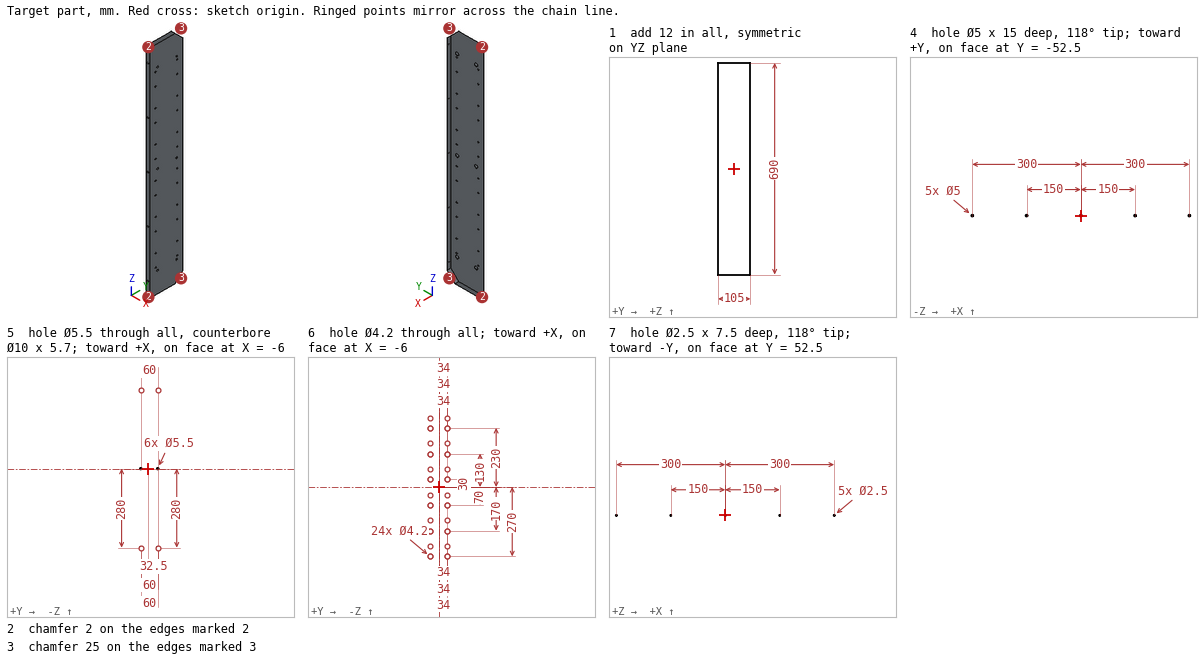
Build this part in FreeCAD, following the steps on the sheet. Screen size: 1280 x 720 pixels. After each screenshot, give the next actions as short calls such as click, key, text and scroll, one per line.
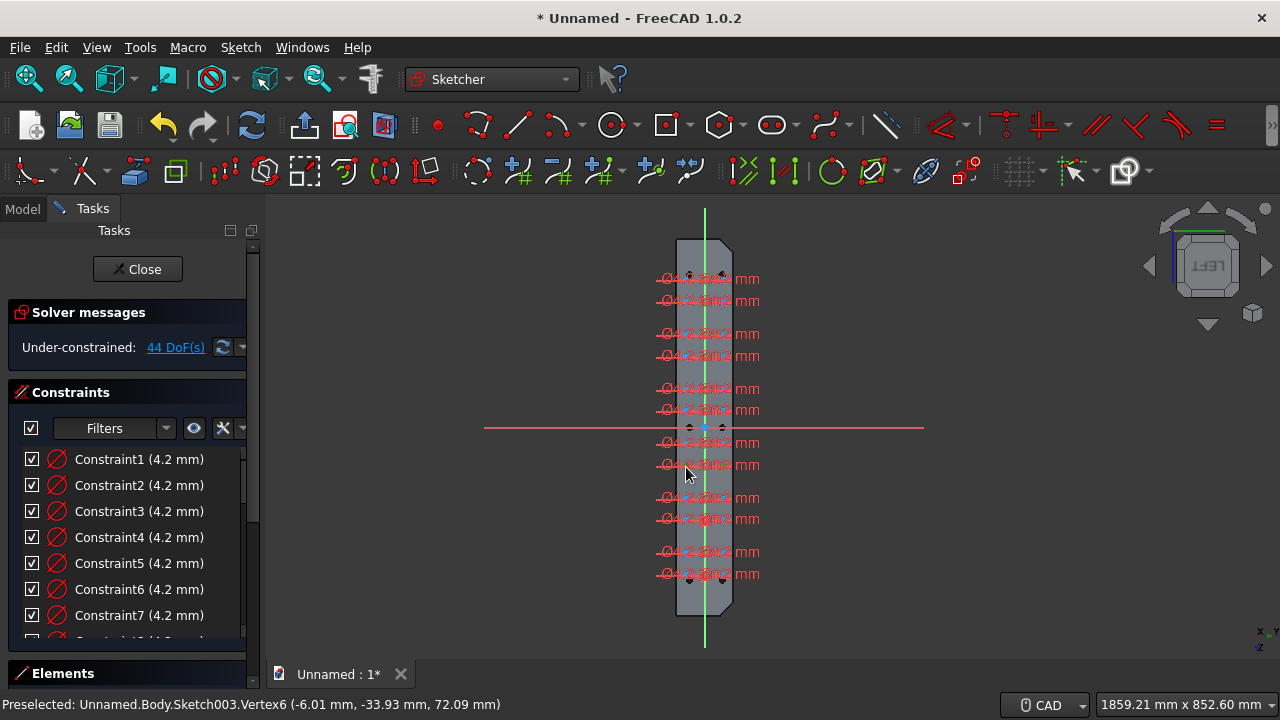
click(705, 602)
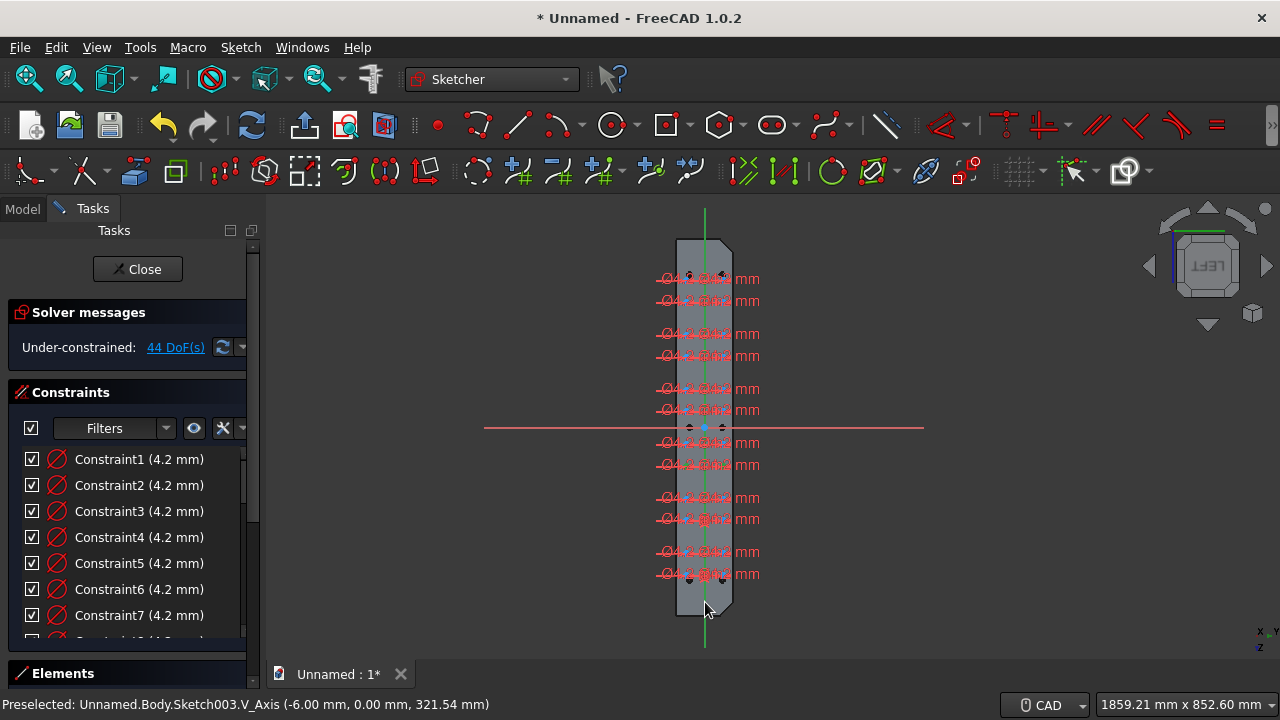
key(s)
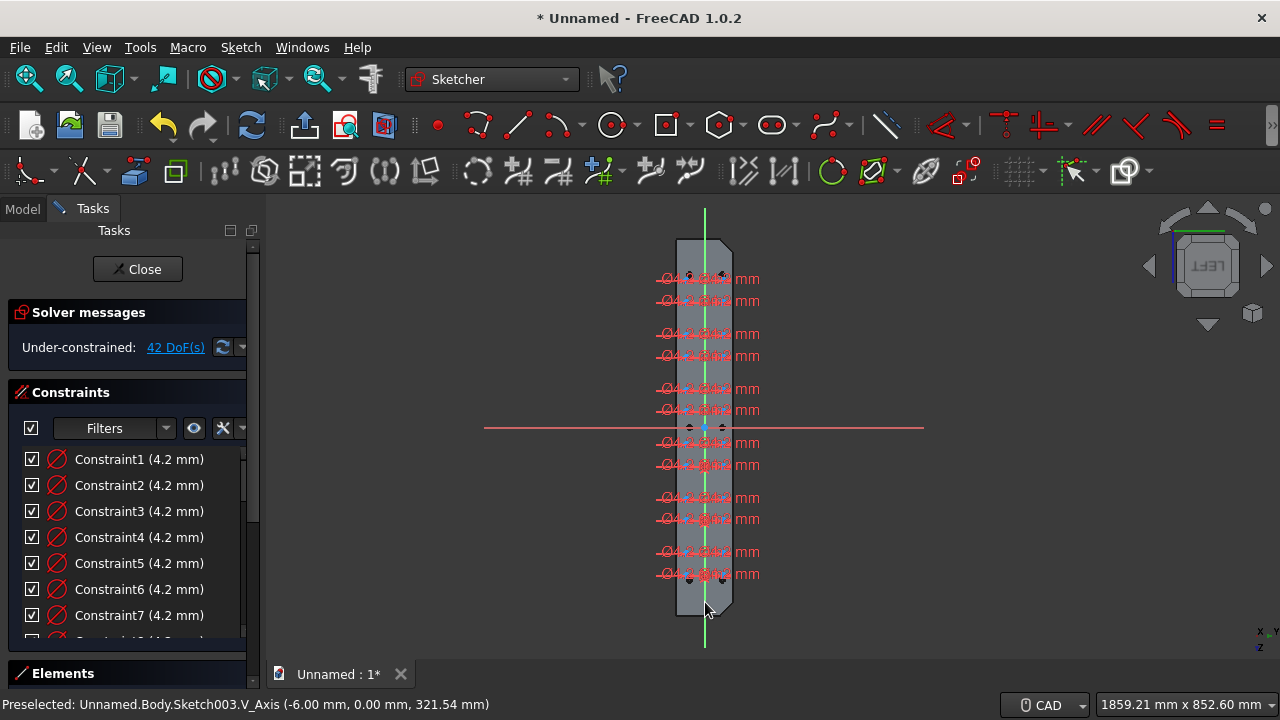
click(723, 412)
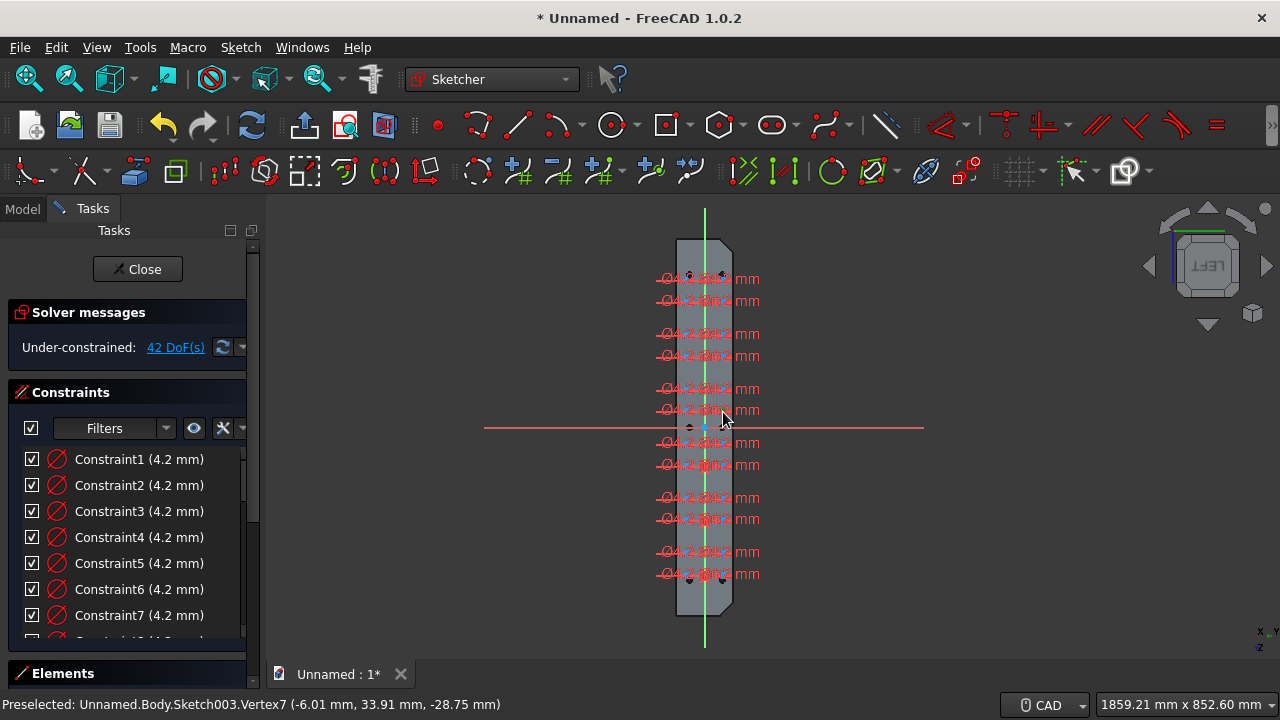
click(686, 412)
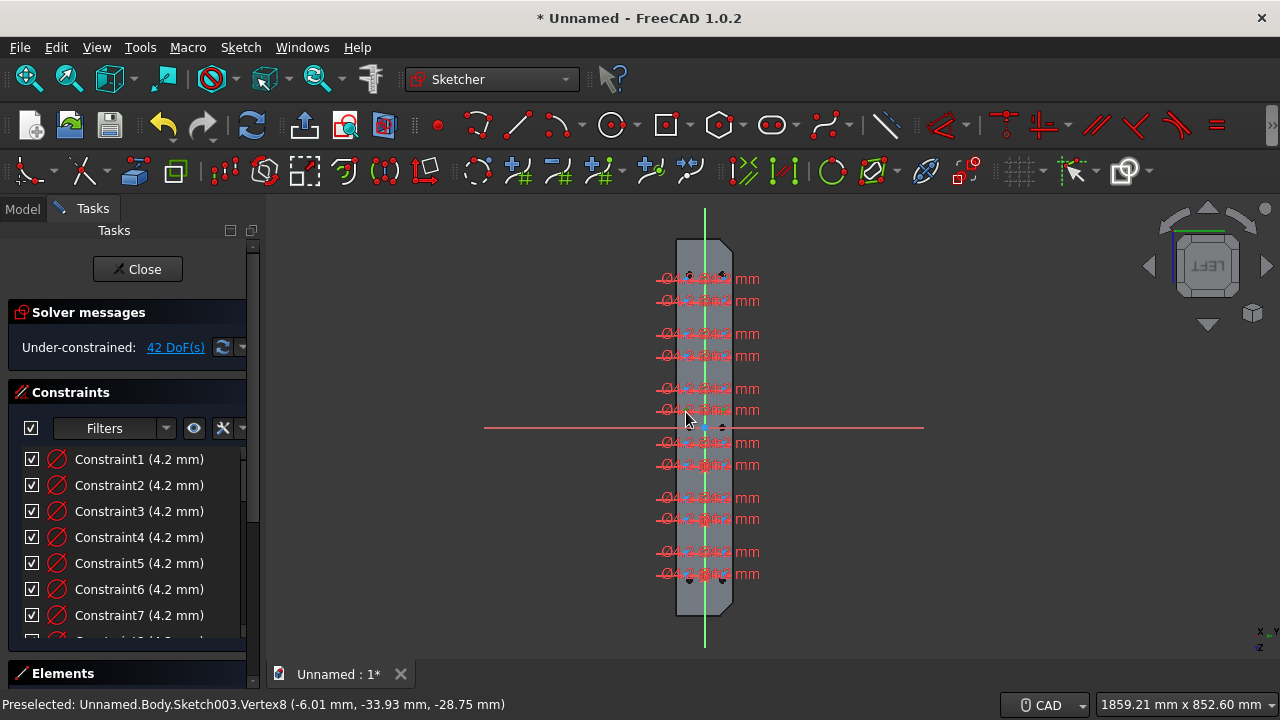
click(705, 602)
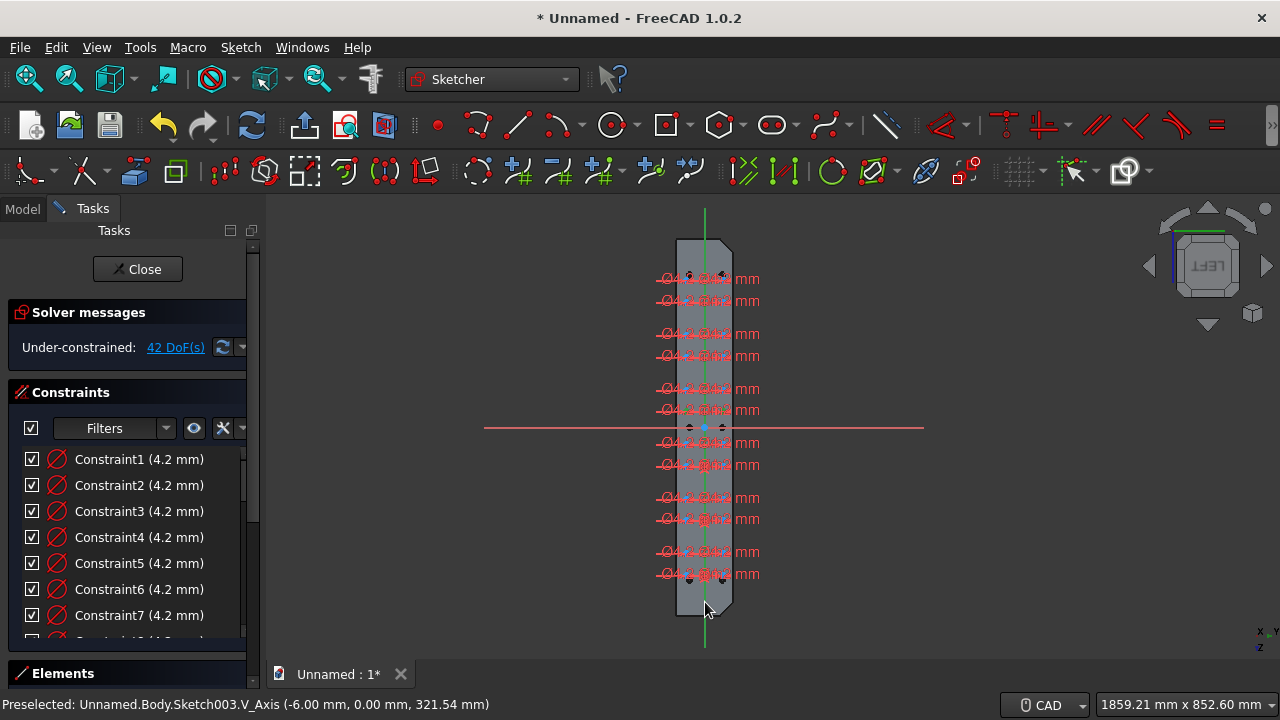
key(s)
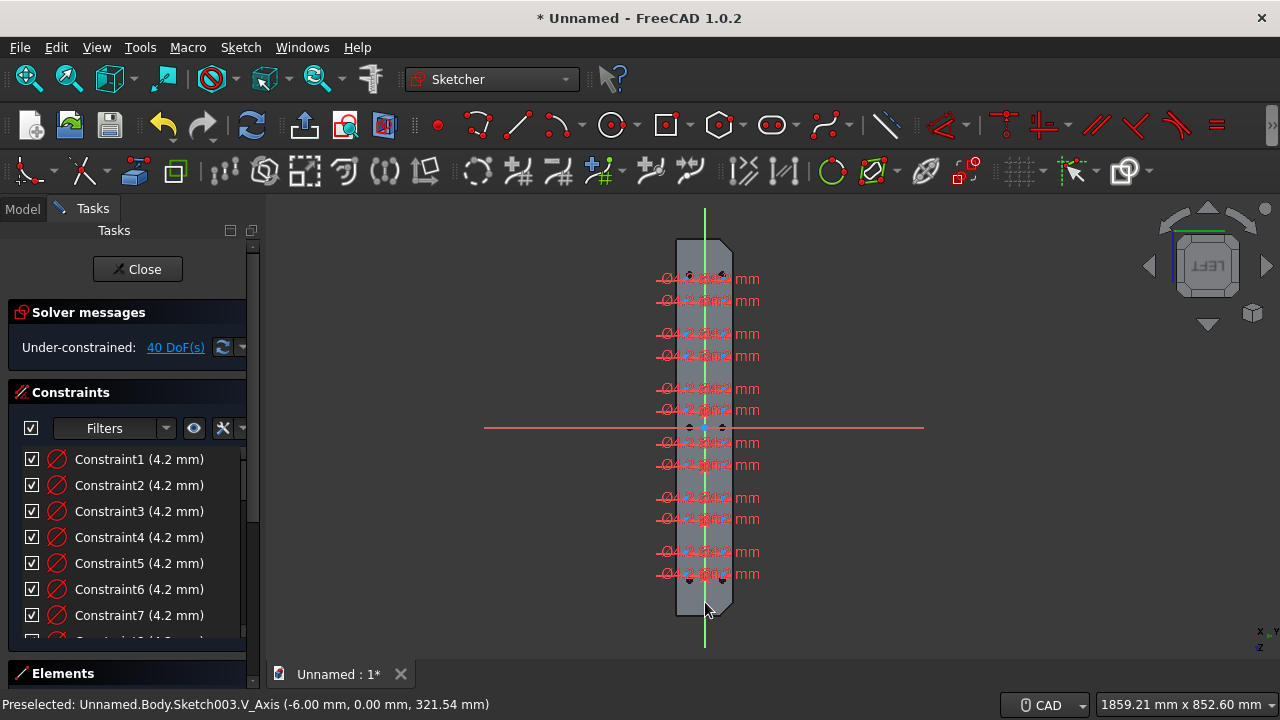
click(723, 358)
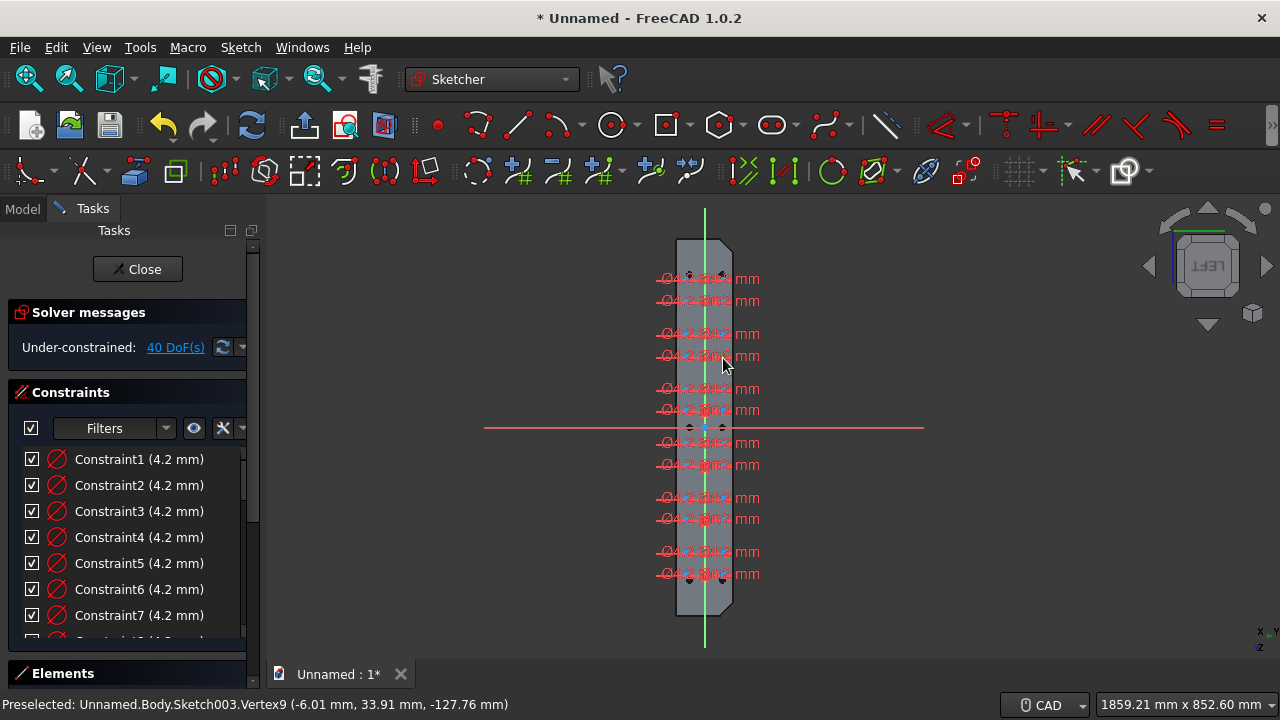
click(686, 358)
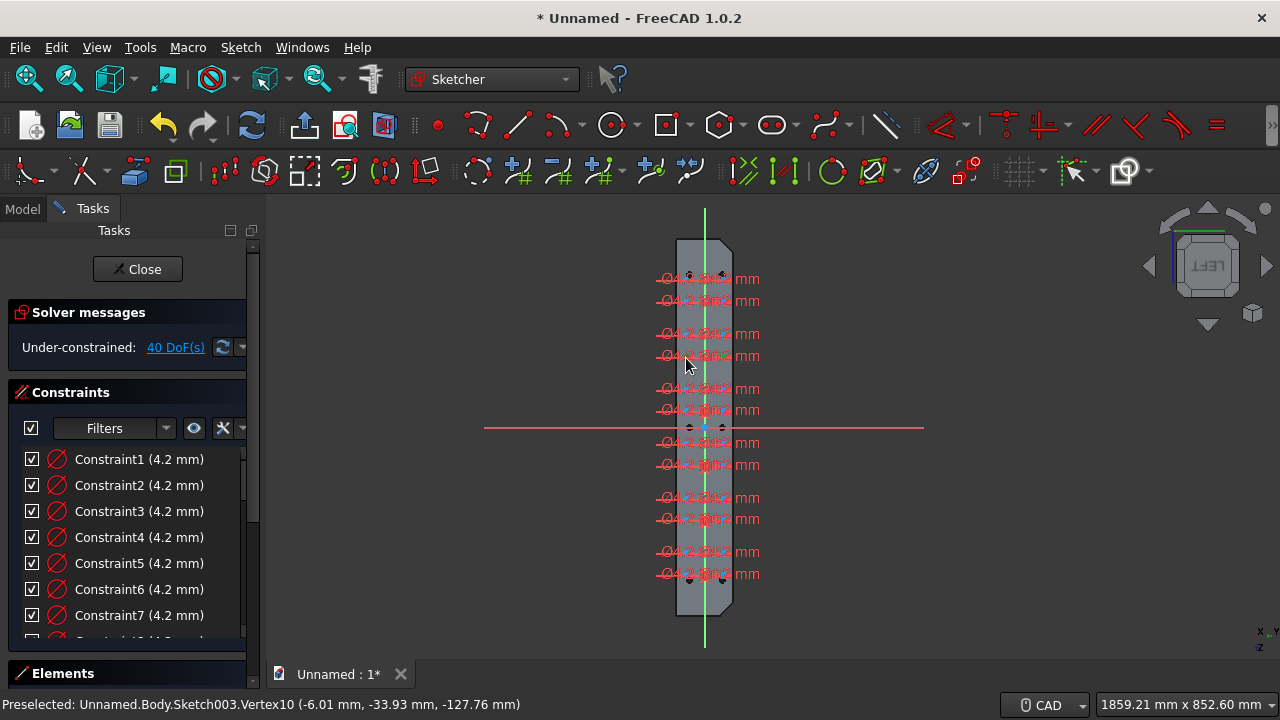
click(705, 602)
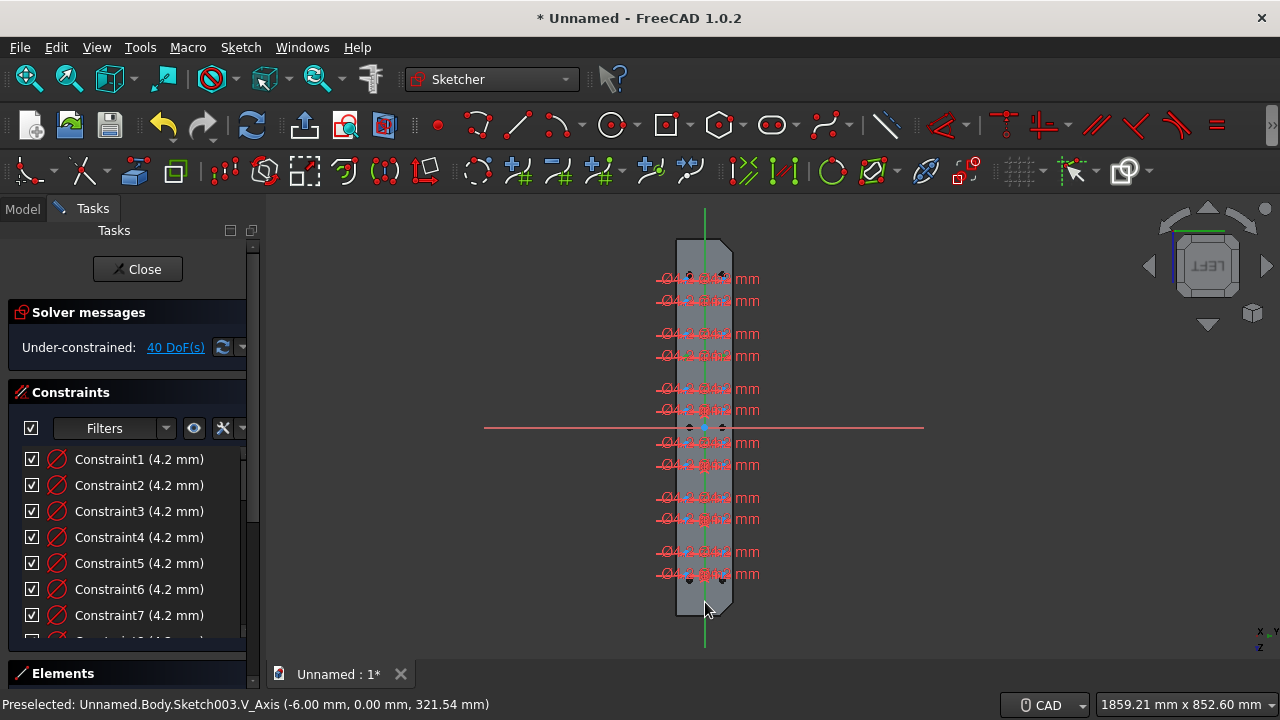
key(s)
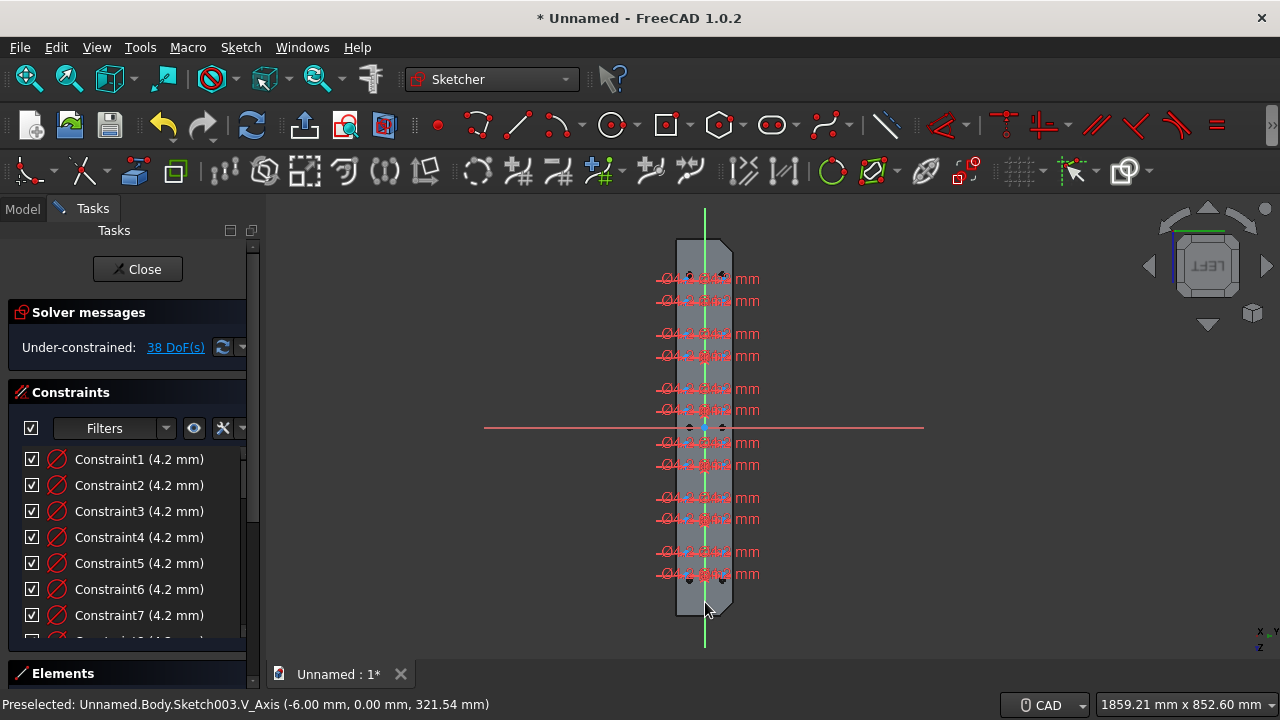
click(686, 358)